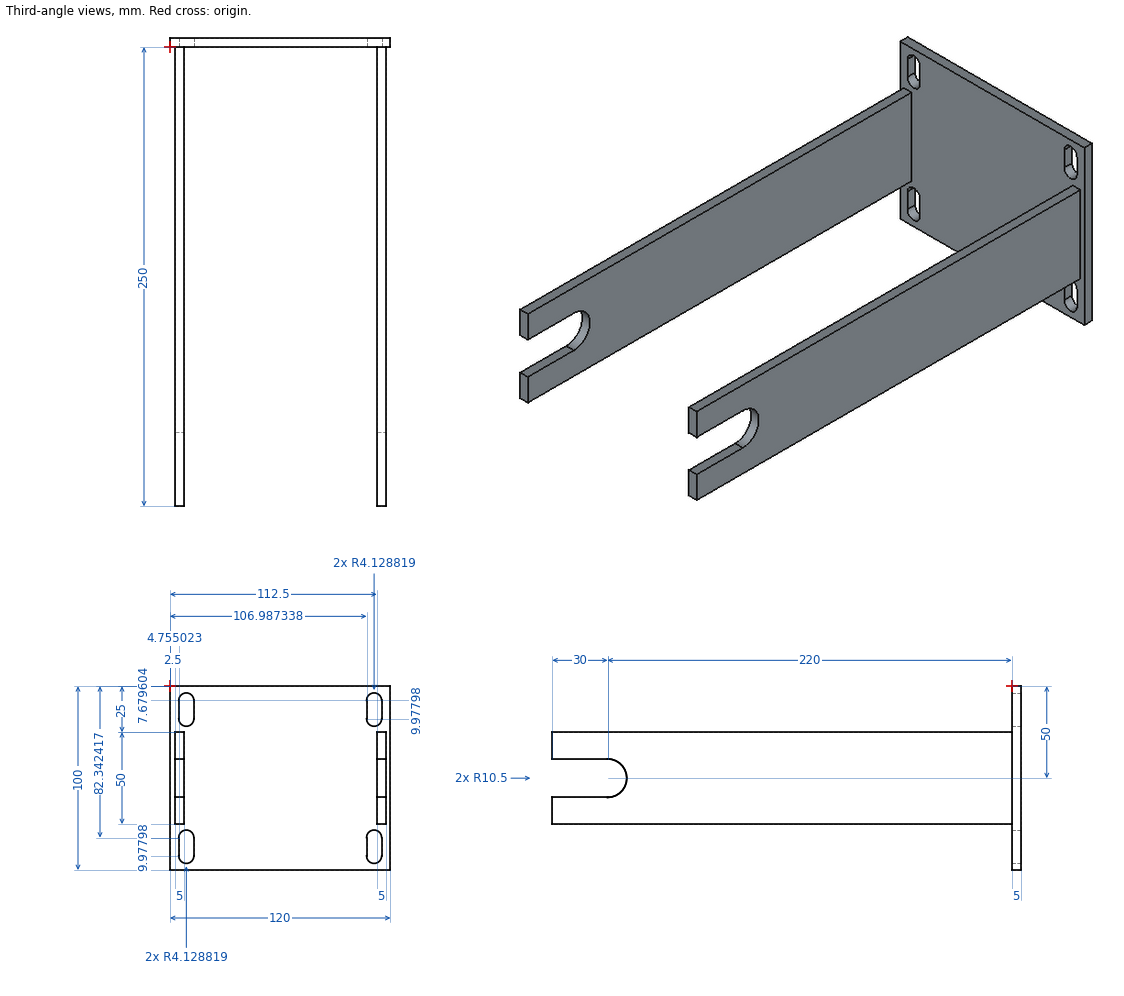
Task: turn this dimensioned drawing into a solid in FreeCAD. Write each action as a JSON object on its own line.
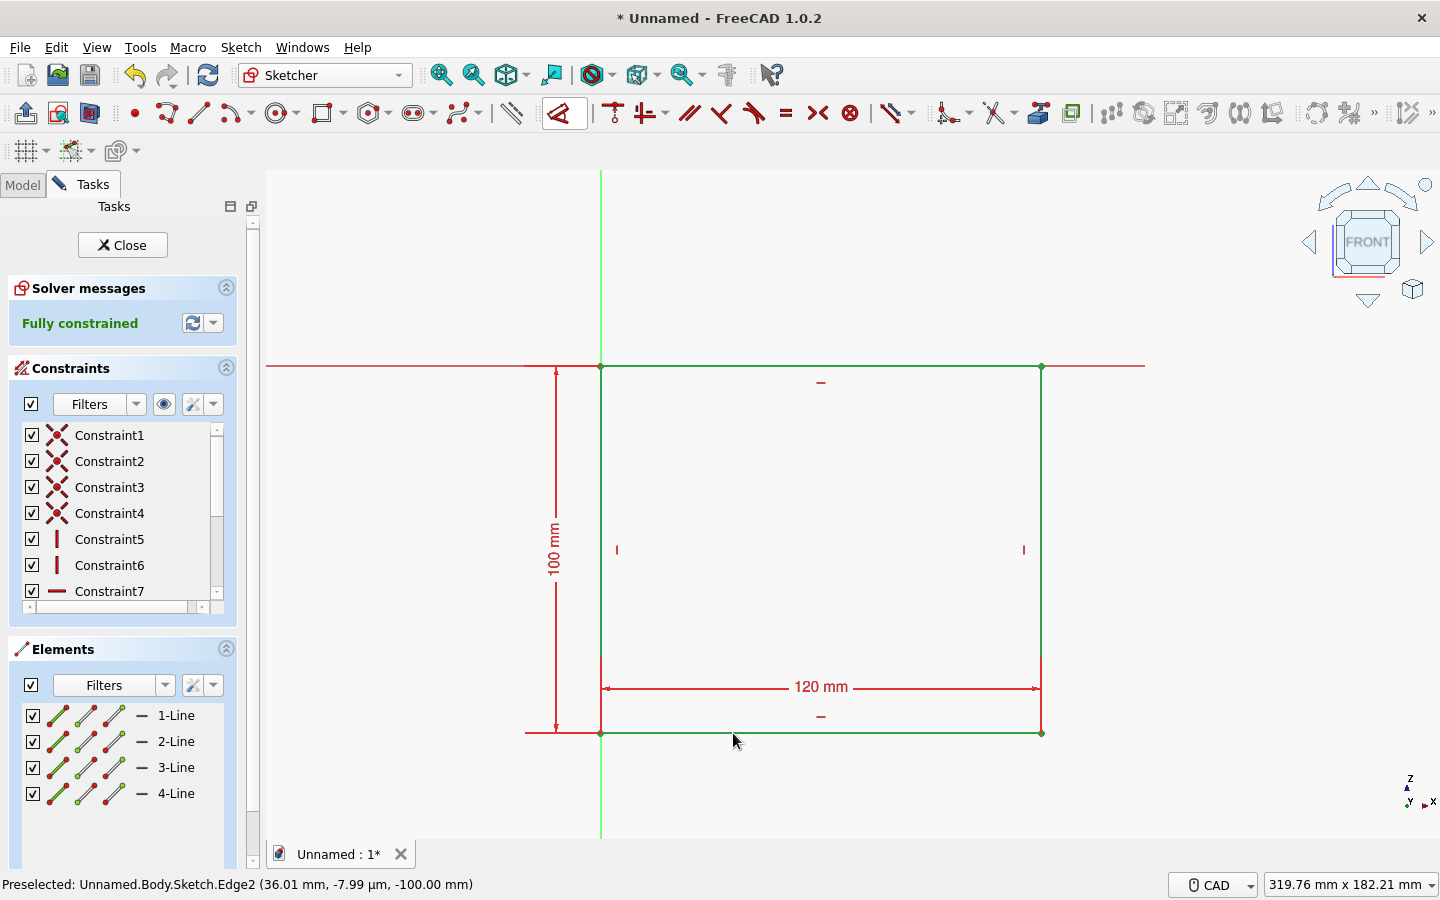
{"action": "left_click", "coordinate": [123, 245]}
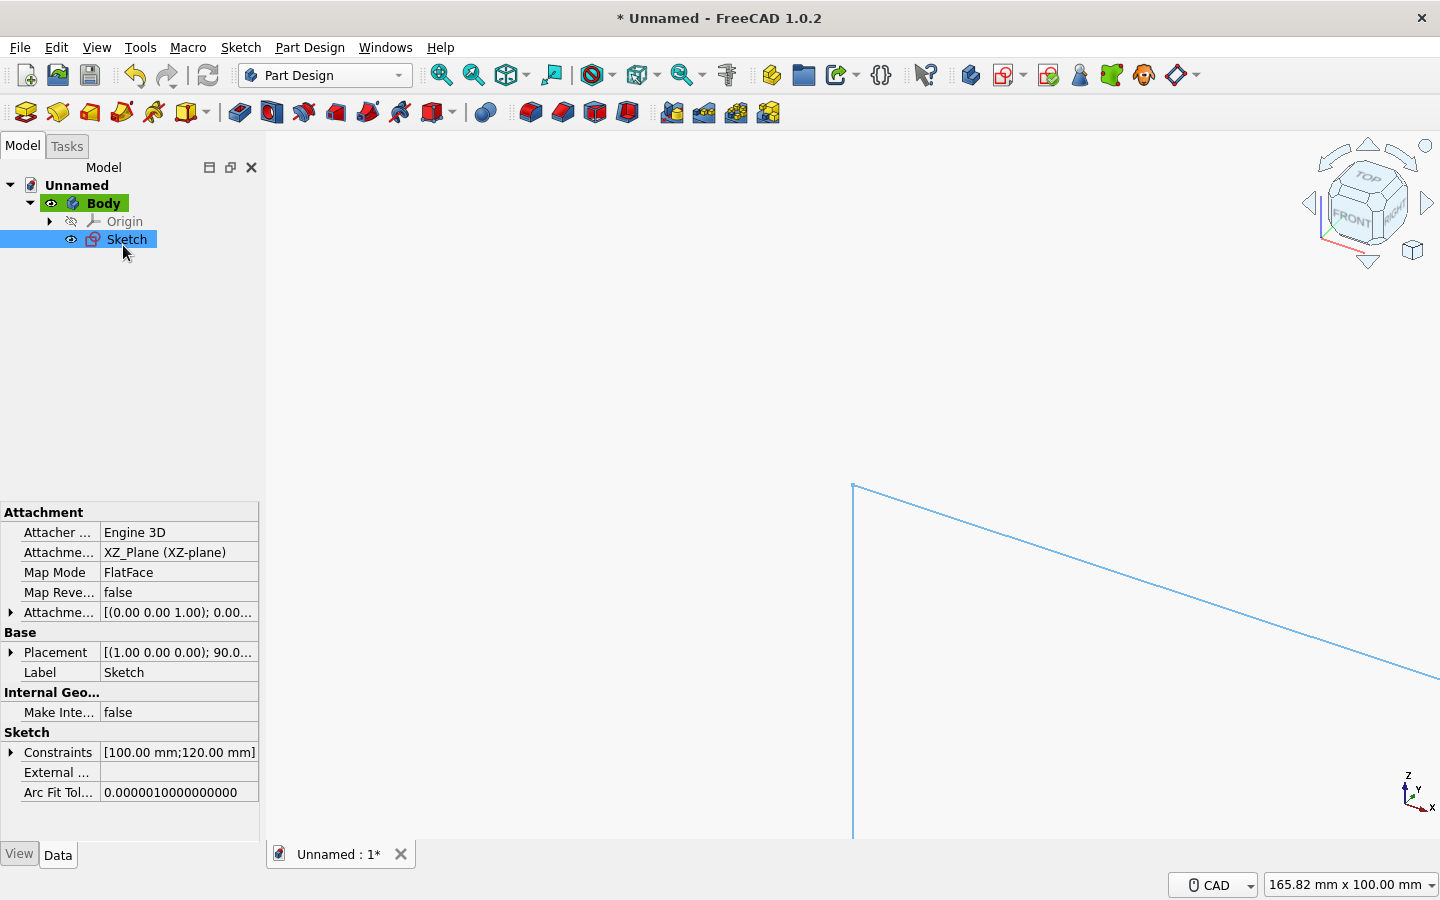
{"action": "left_click", "coordinate": [26, 112]}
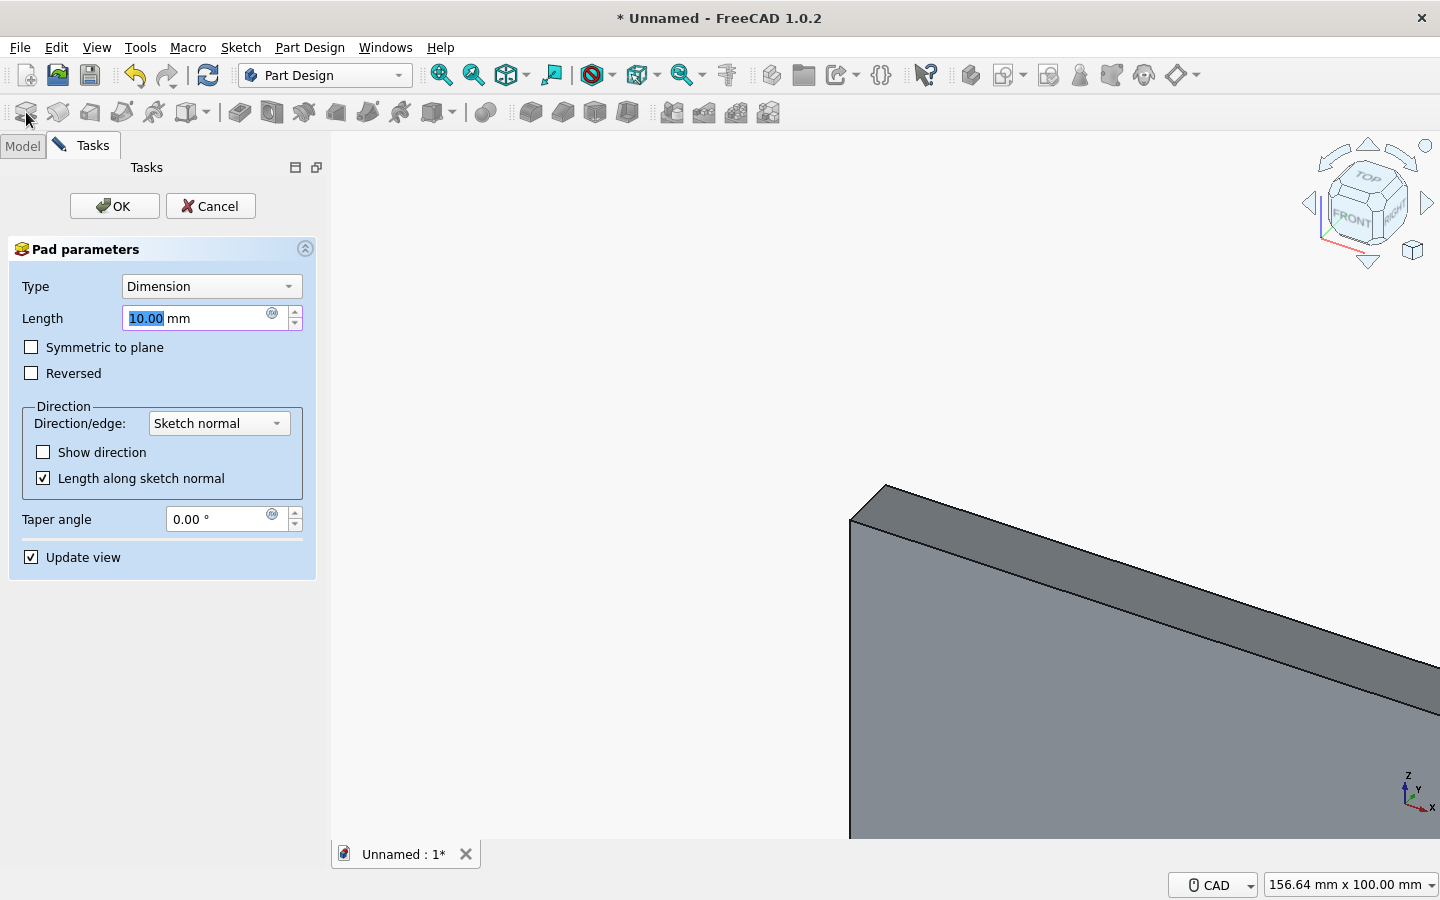
{"action": "type", "text": "5"}
{"action": "key", "text": "Tab"}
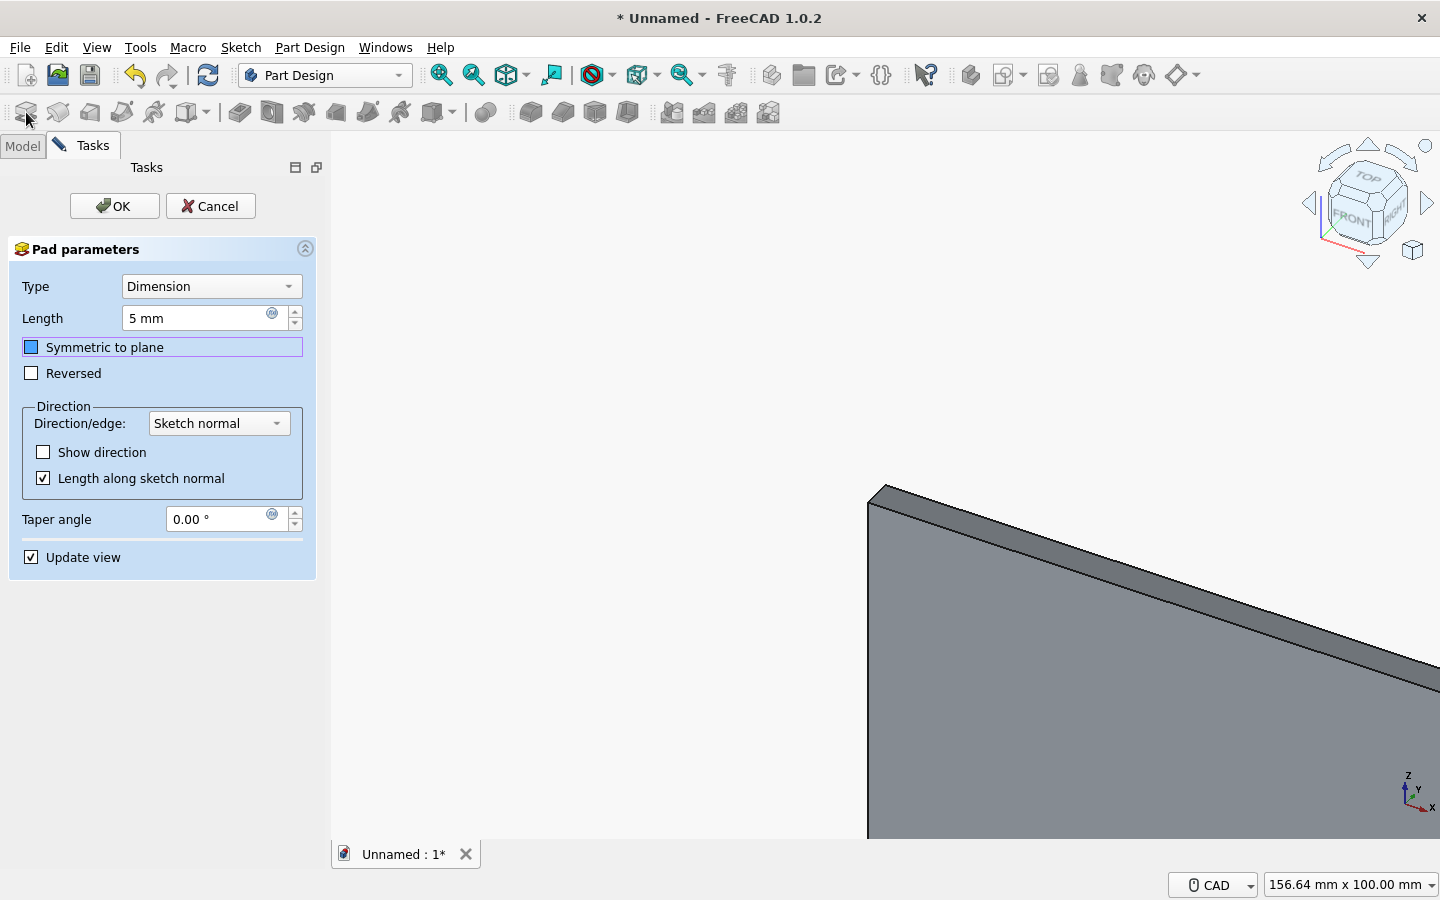
{"action": "left_click", "coordinate": [30, 373]}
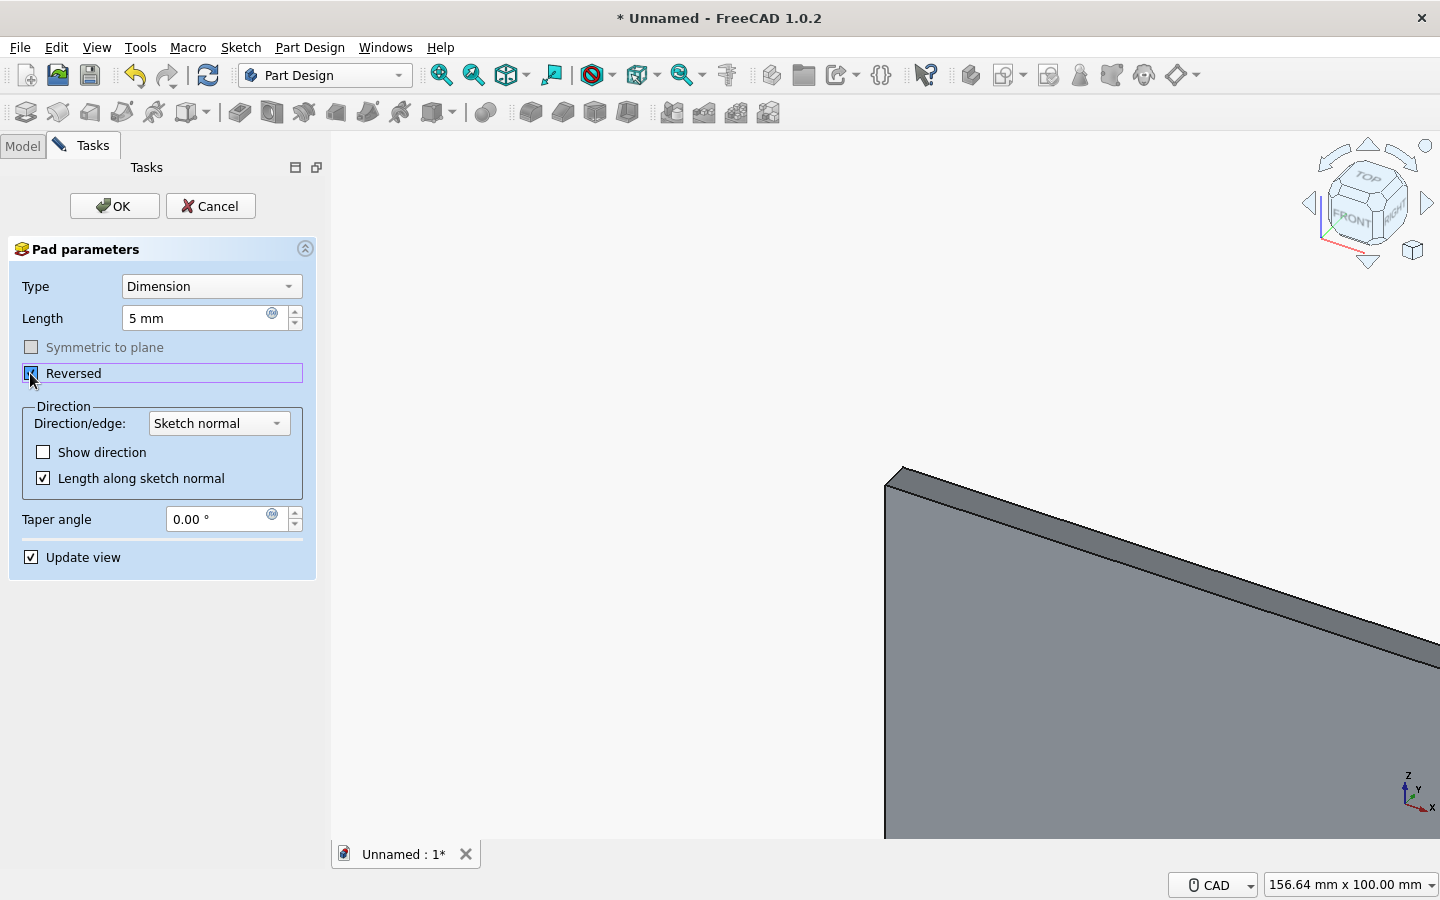
{"action": "left_click", "coordinate": [115, 206]}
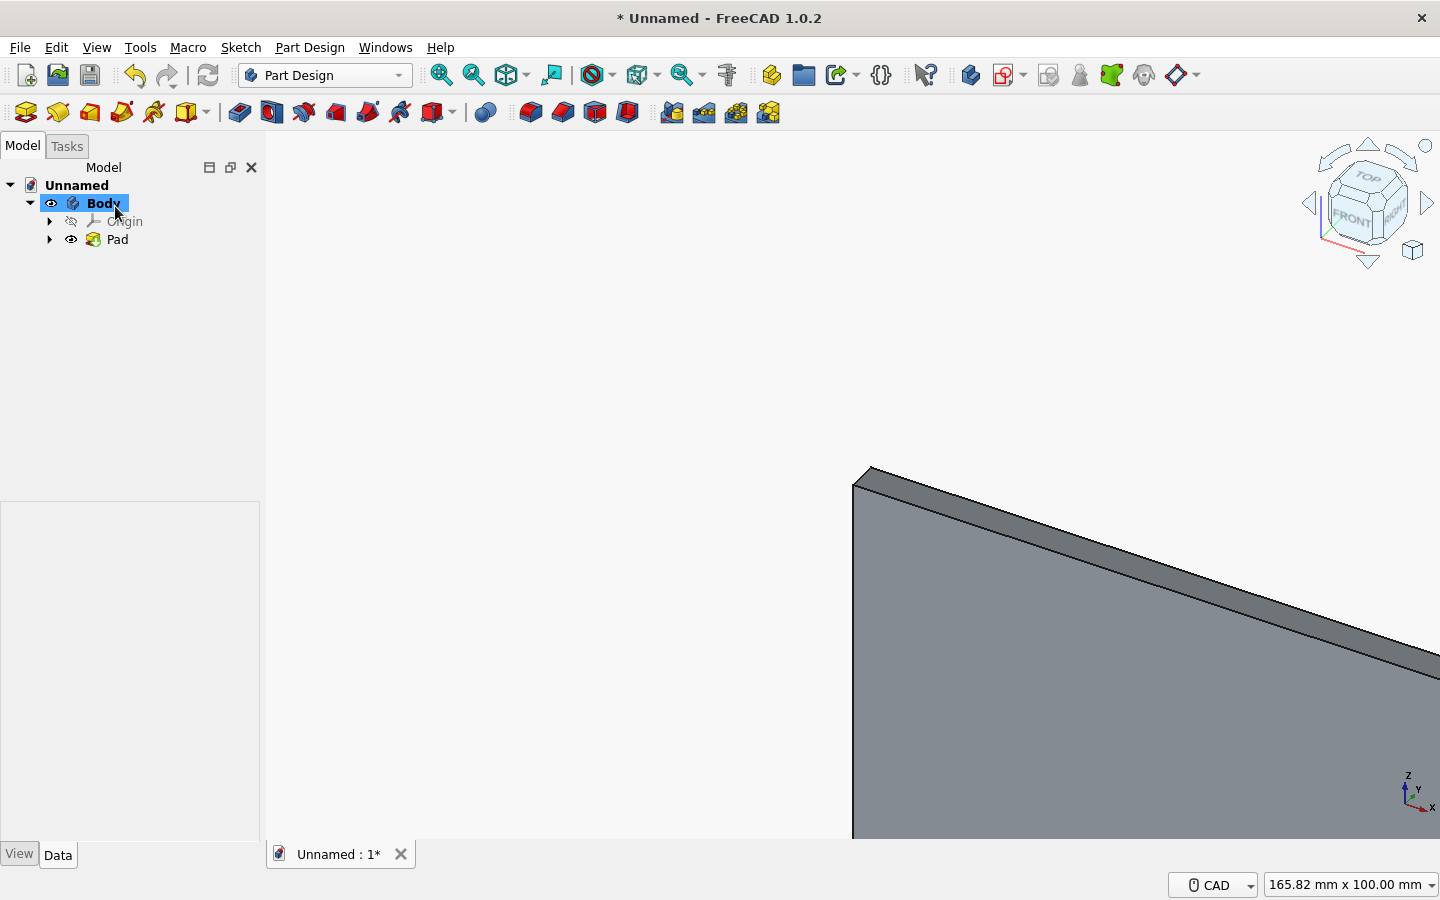
{"action": "left_click", "coordinate": [442, 76]}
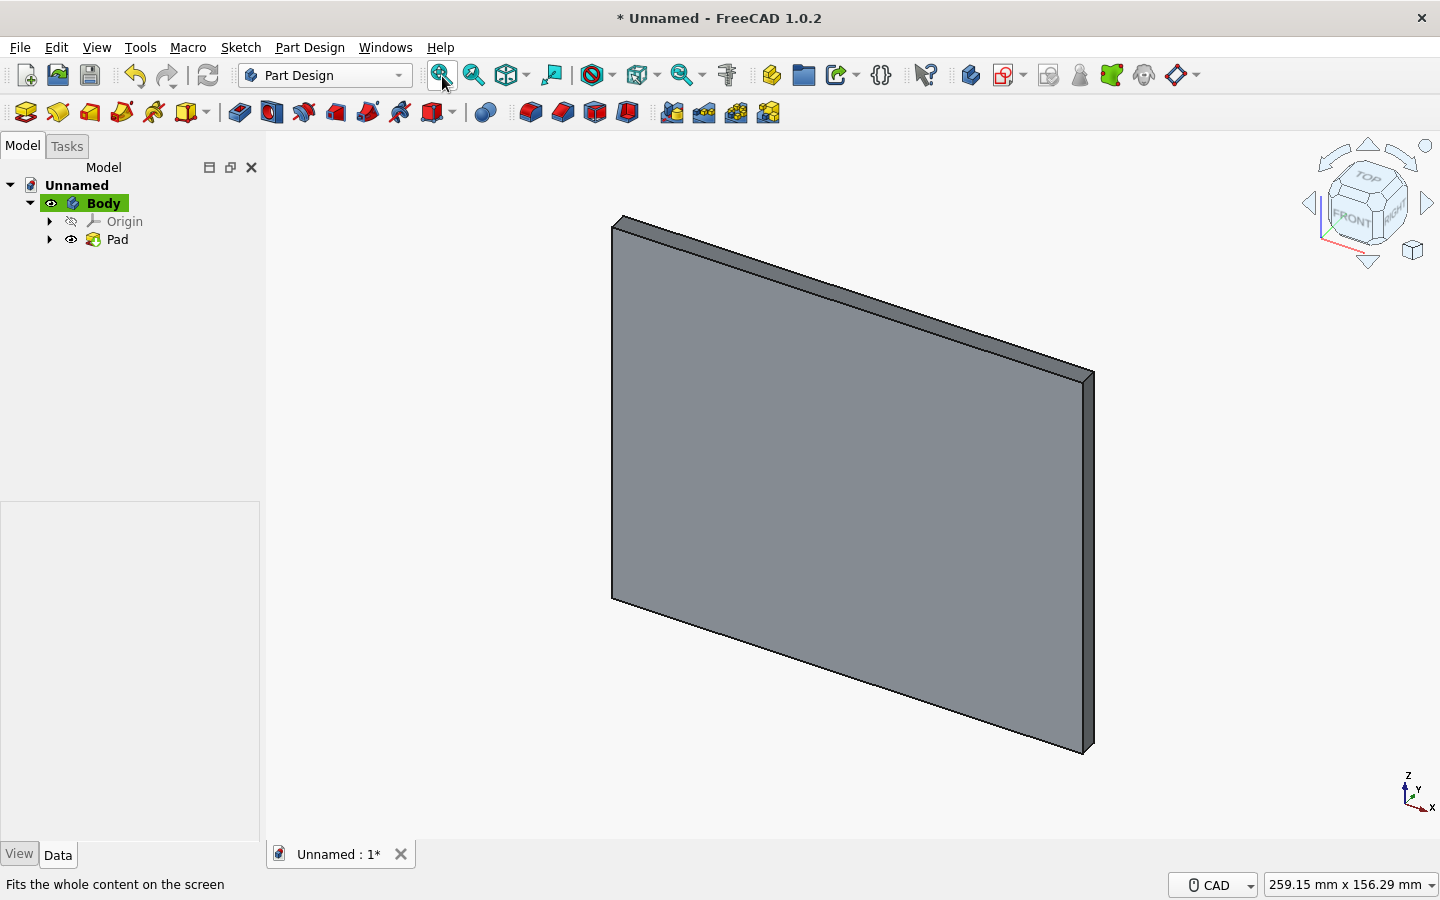
{"action": "key", "text": "4"}